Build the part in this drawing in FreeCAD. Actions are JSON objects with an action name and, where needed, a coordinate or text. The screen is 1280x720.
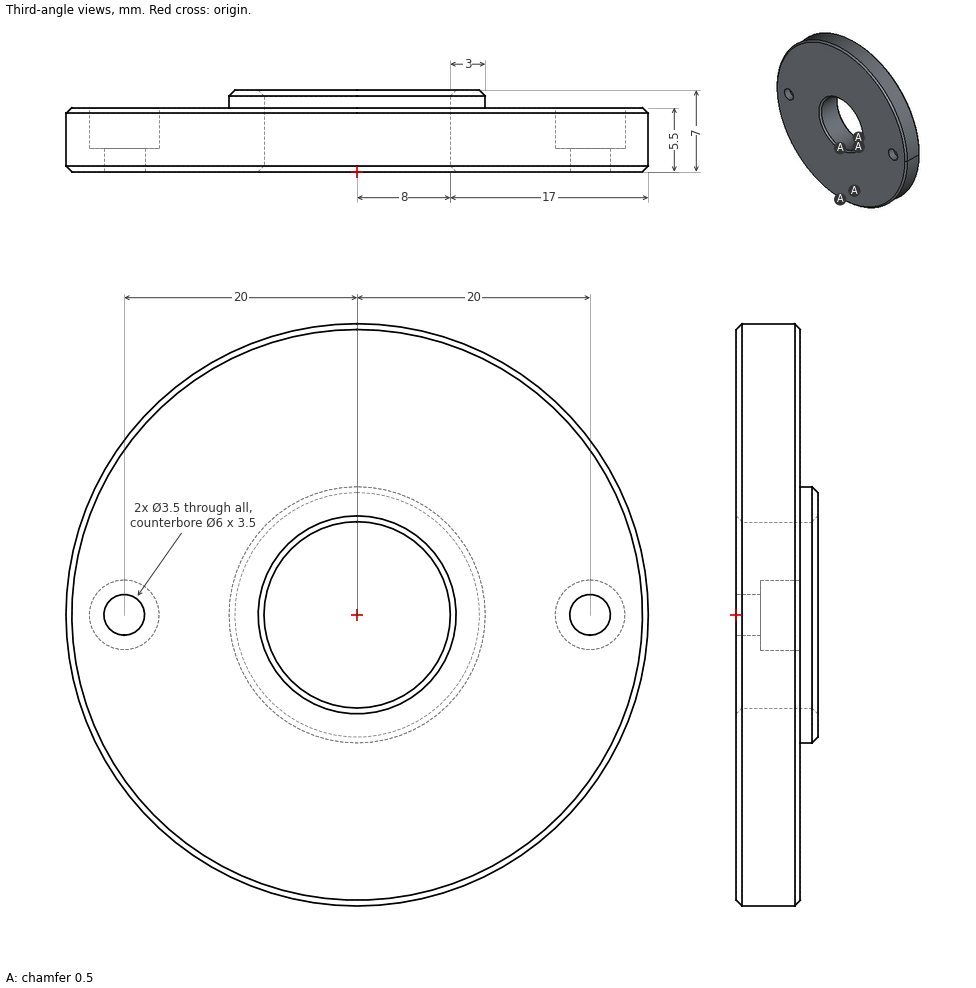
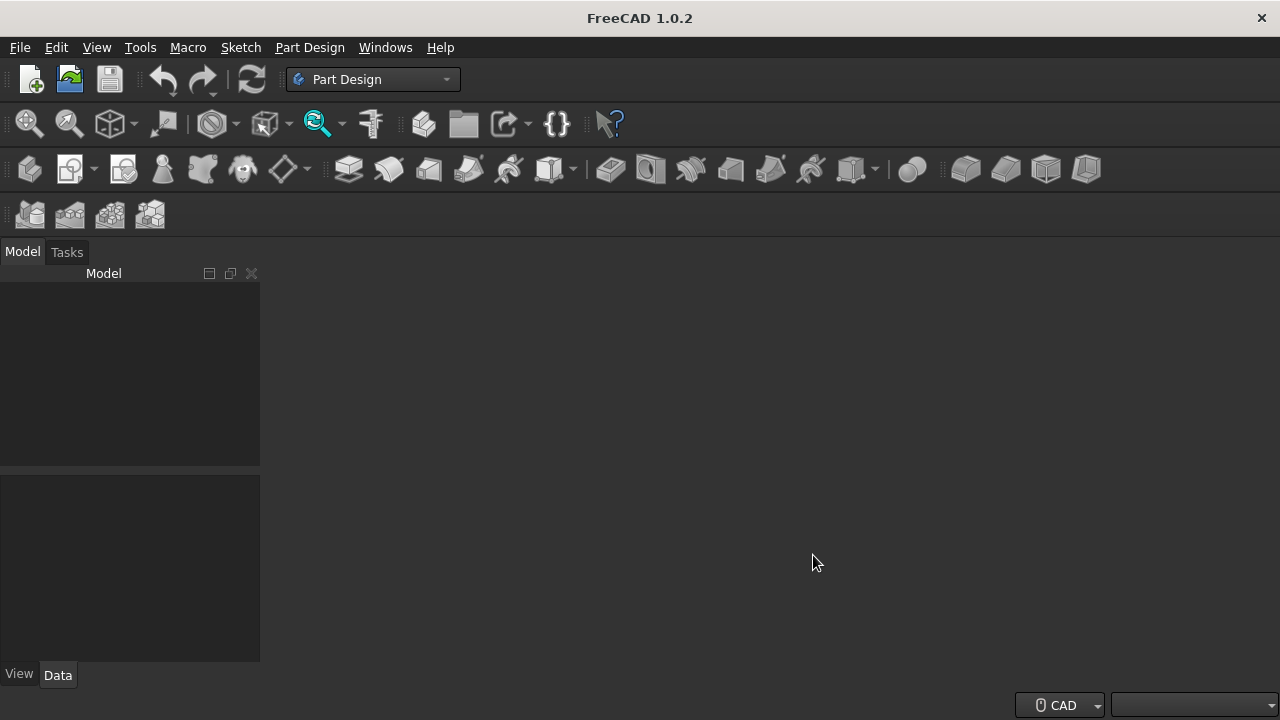
{"action": "left_click", "coordinate": [30, 80]}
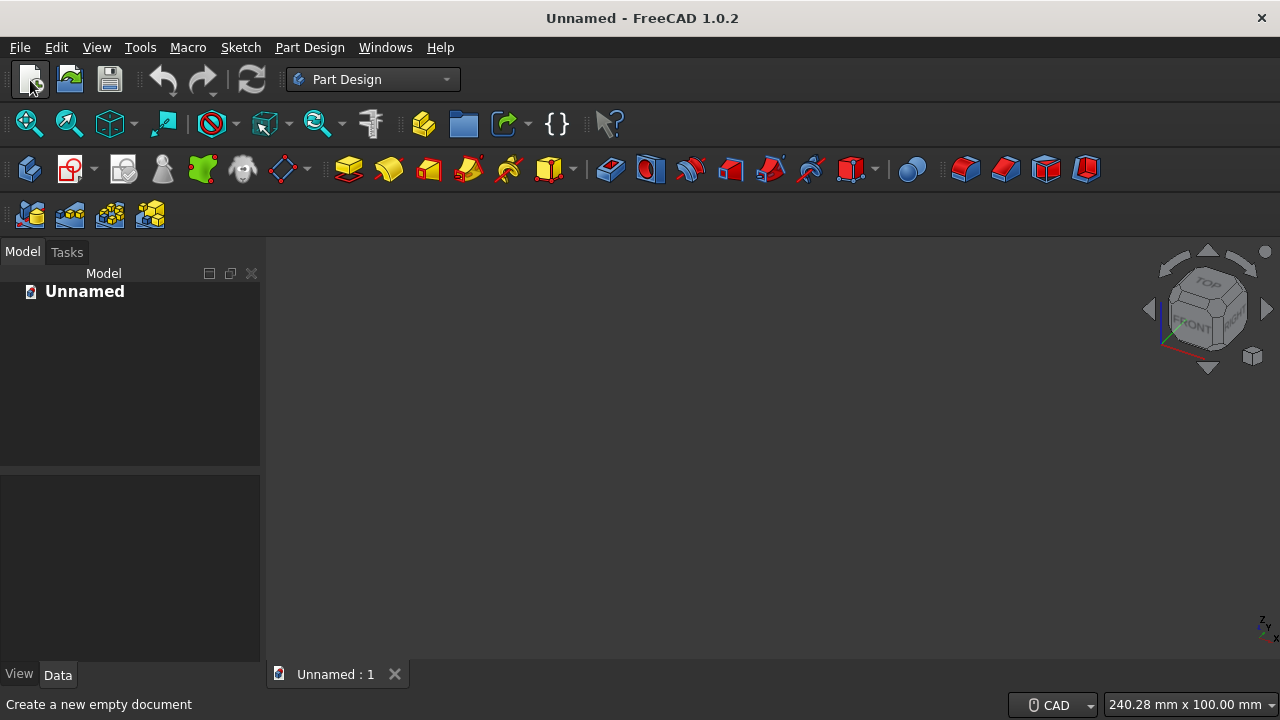
{"action": "left_click", "coordinate": [70, 170]}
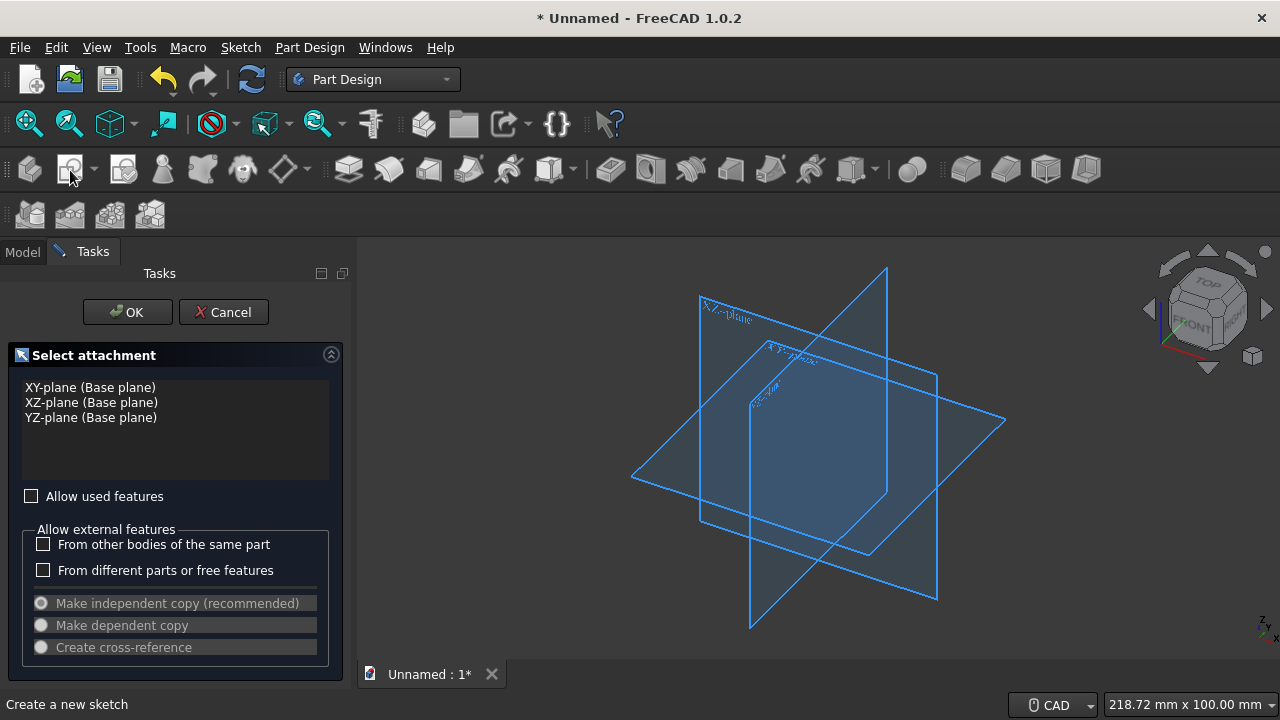
{"action": "left_click", "coordinate": [82, 388]}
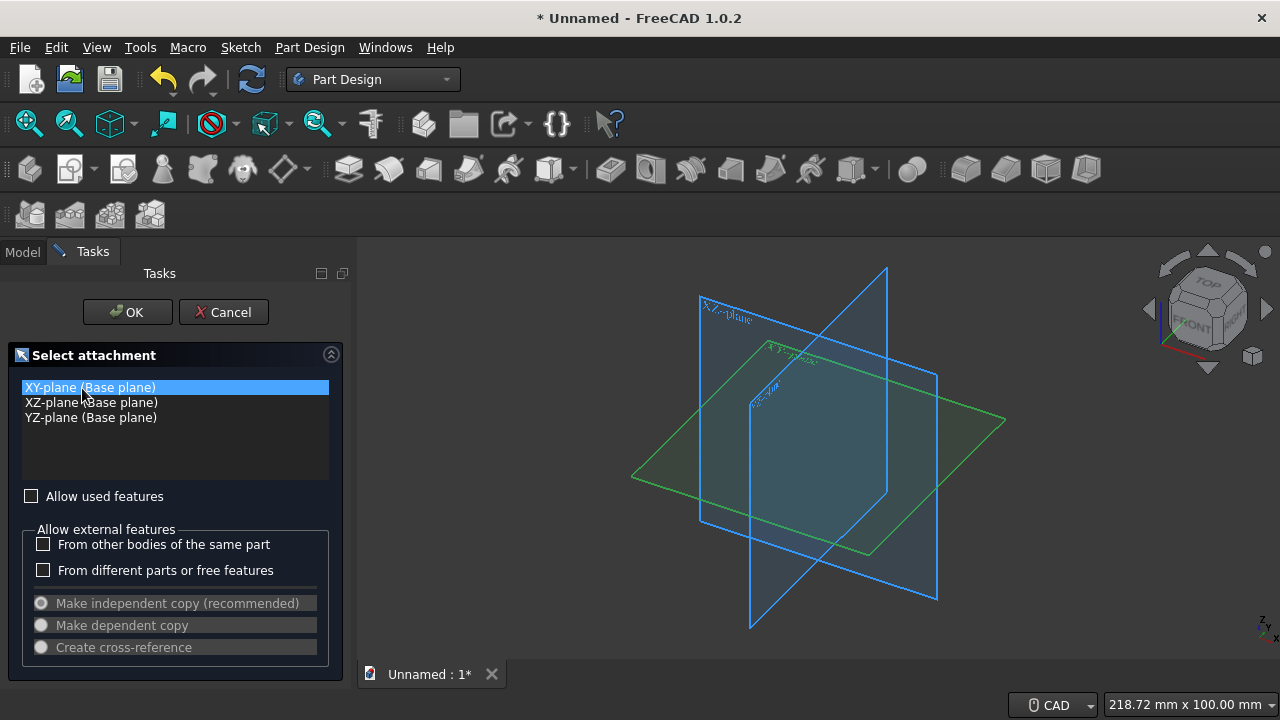
{"action": "left_click", "coordinate": [128, 312]}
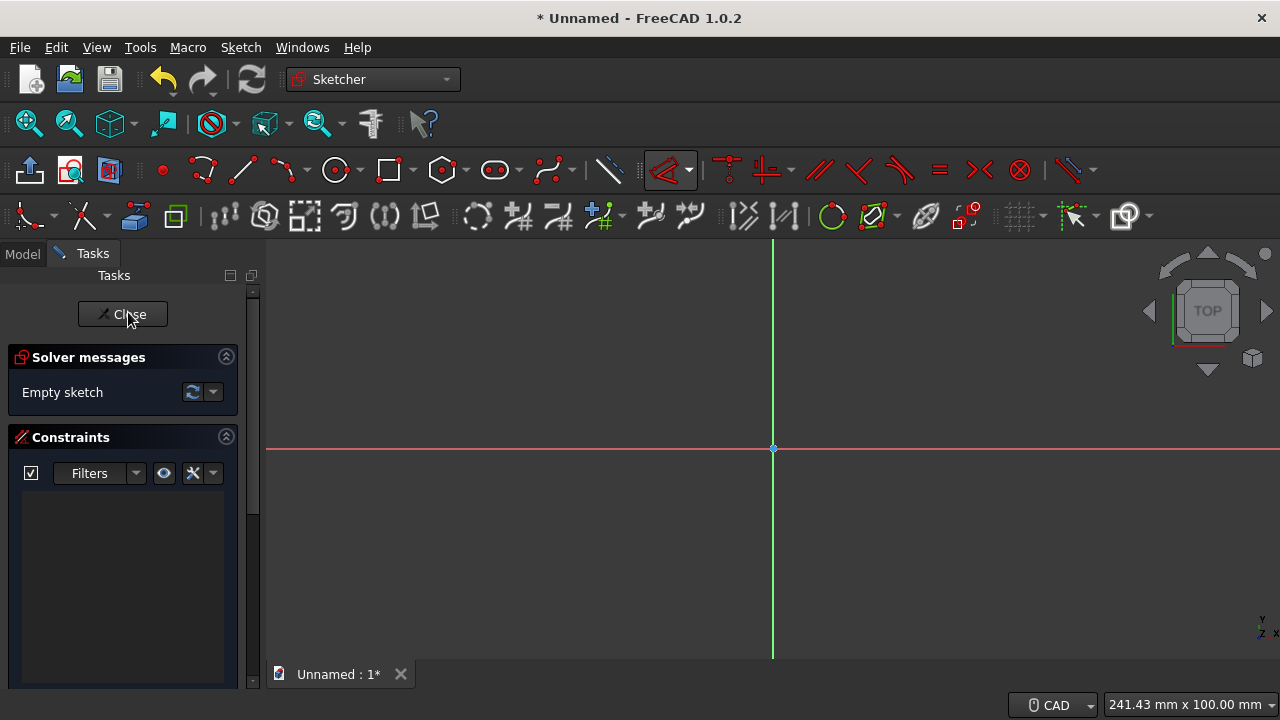
{"action": "scroll", "coordinate": [849, 431], "scroll_direction": "up", "scroll_amount": 9}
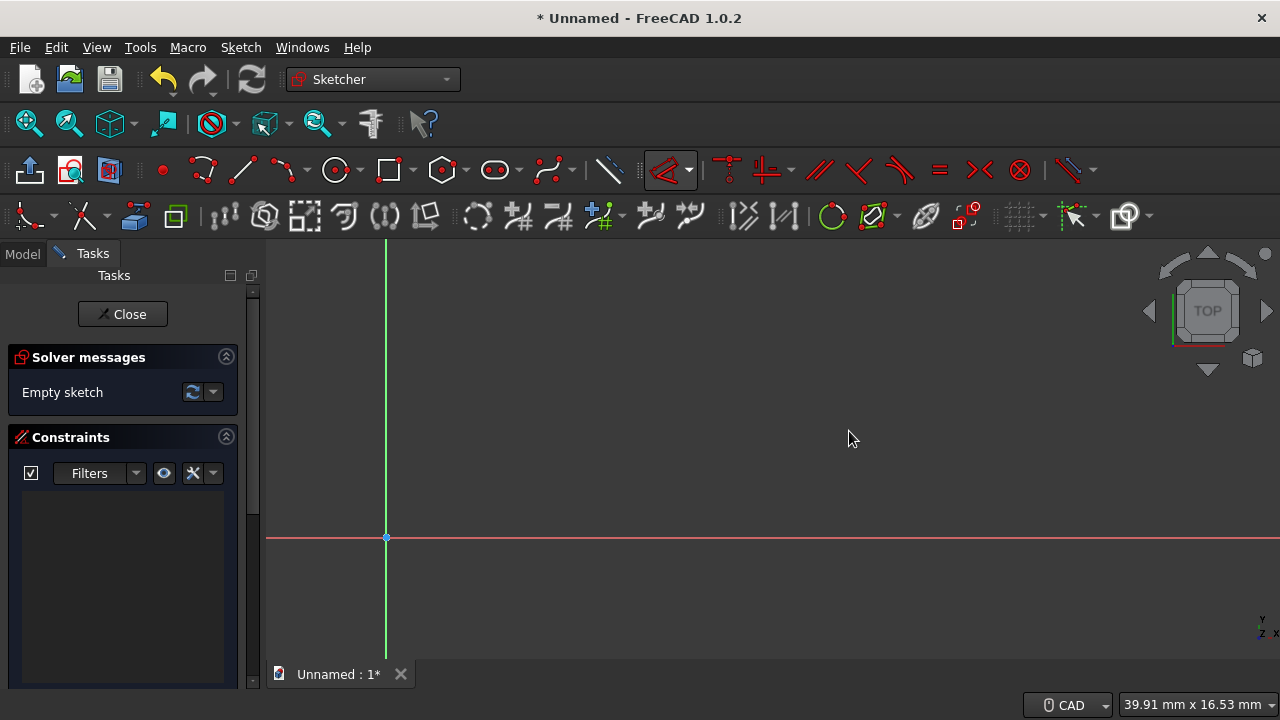
{"action": "key", "text": "g m"}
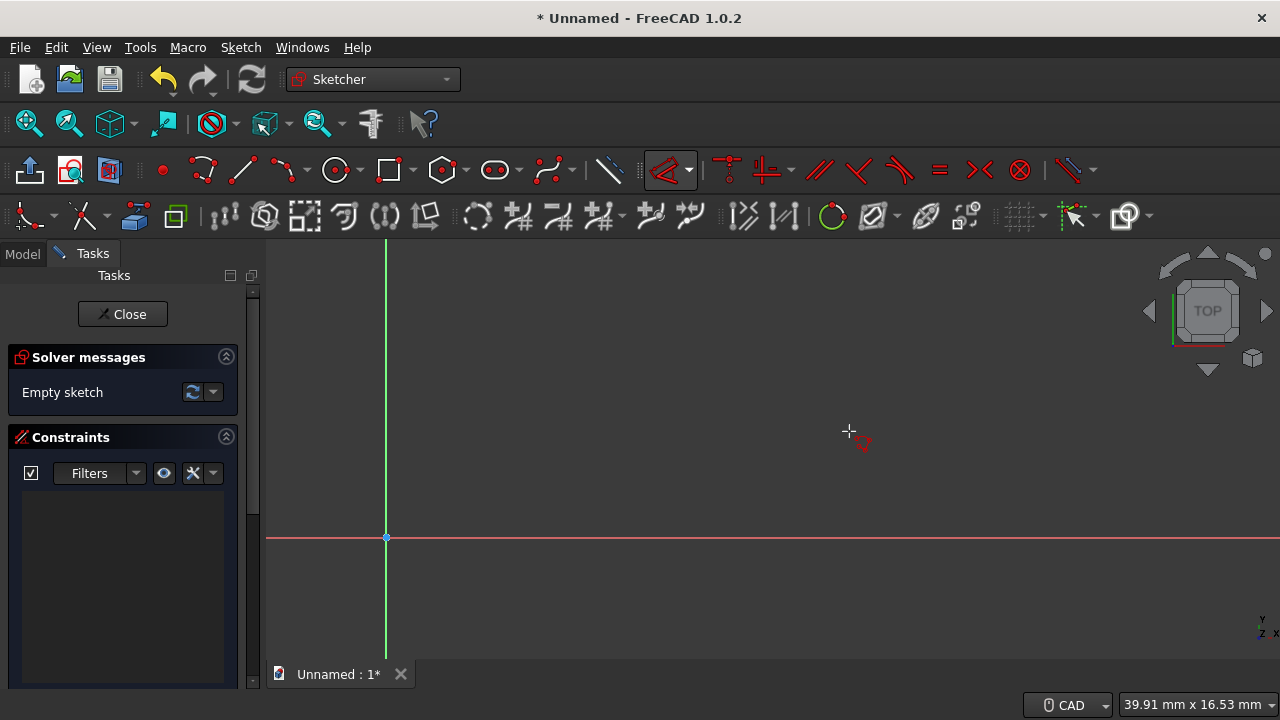
{"action": "left_click", "coordinate": [590, 538]}
{"action": "left_click", "coordinate": [1022, 529]}
{"action": "left_click", "coordinate": [1022, 398]}
{"action": "left_click", "coordinate": [666, 398]}
{"action": "left_click", "coordinate": [666, 360]}
{"action": "left_click", "coordinate": [590, 360]}
{"action": "left_click", "coordinate": [590, 538]}
{"action": "key", "text": "Escape"}
{"action": "key", "text": "Escape"}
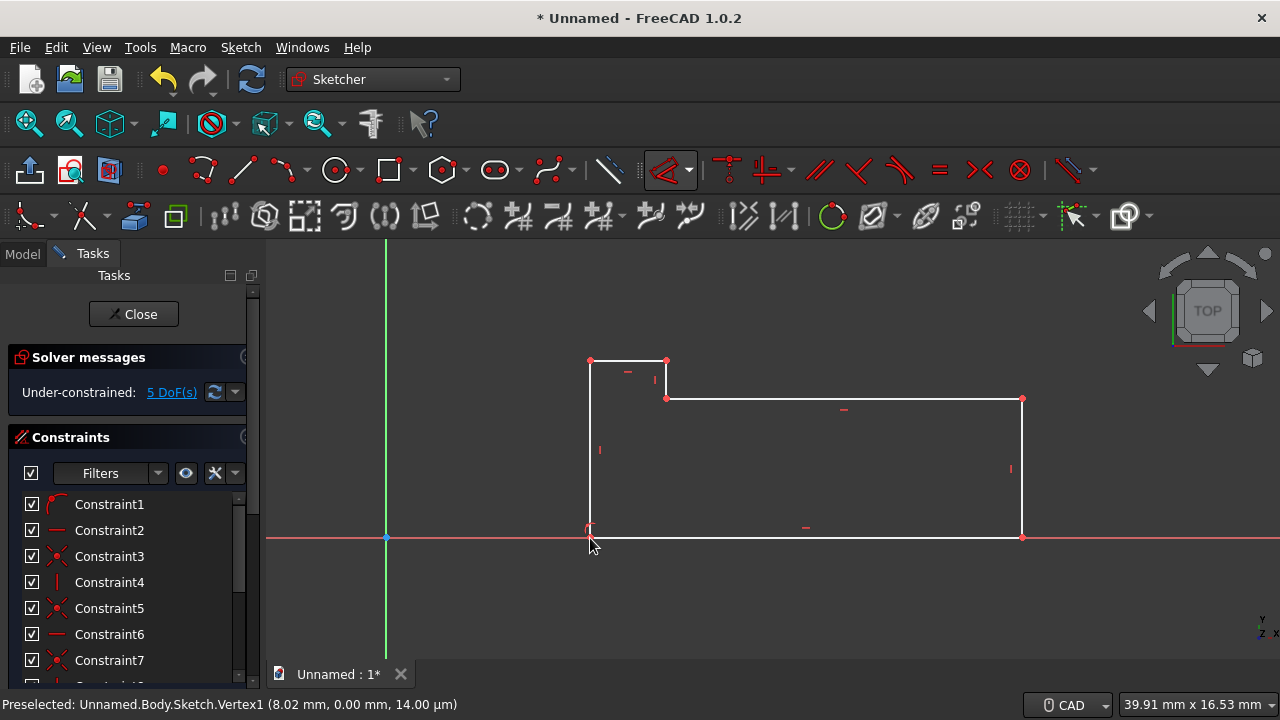
{"action": "left_click", "coordinate": [643, 361]}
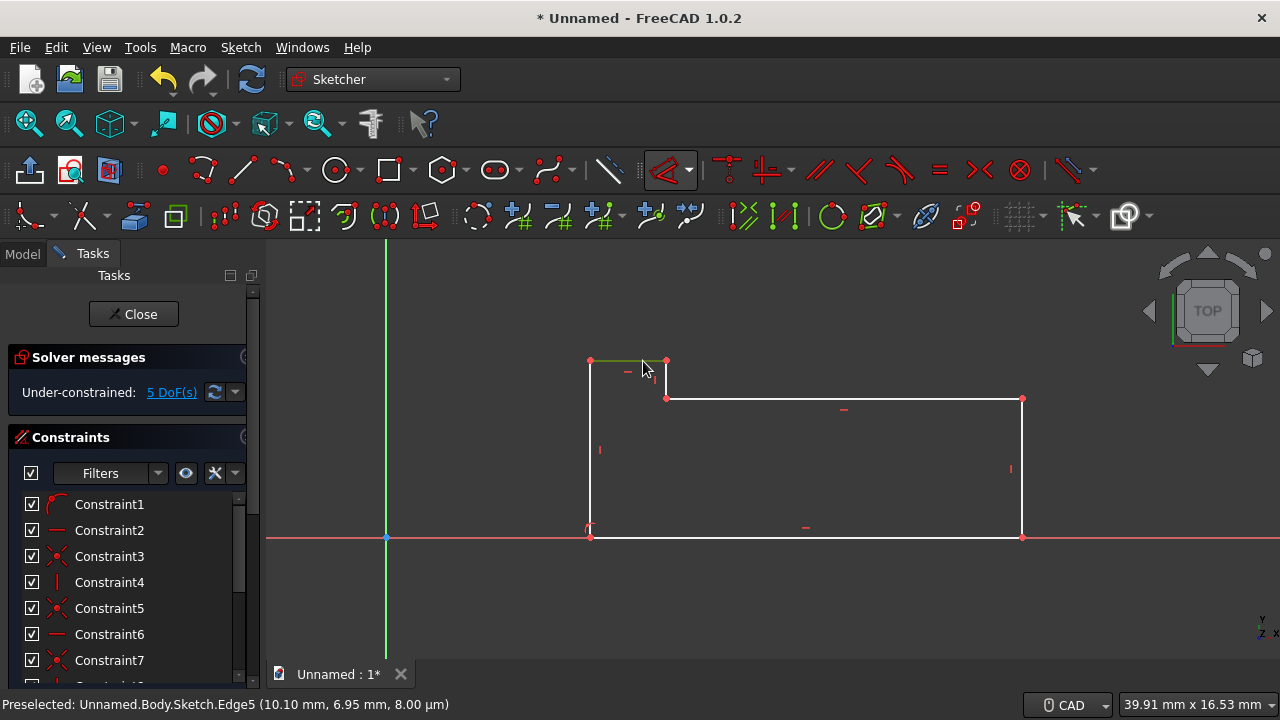
{"action": "key", "text": "l"}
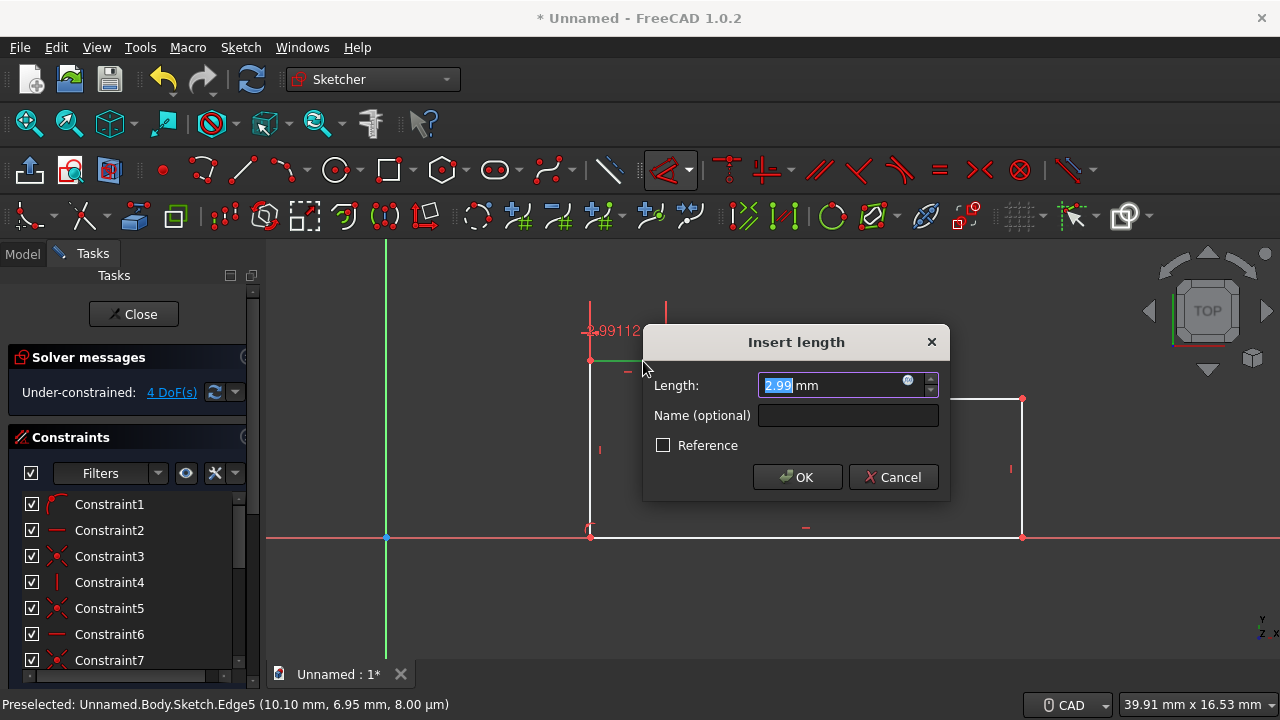
{"action": "type", "text": "3"}
{"action": "key", "text": "Return"}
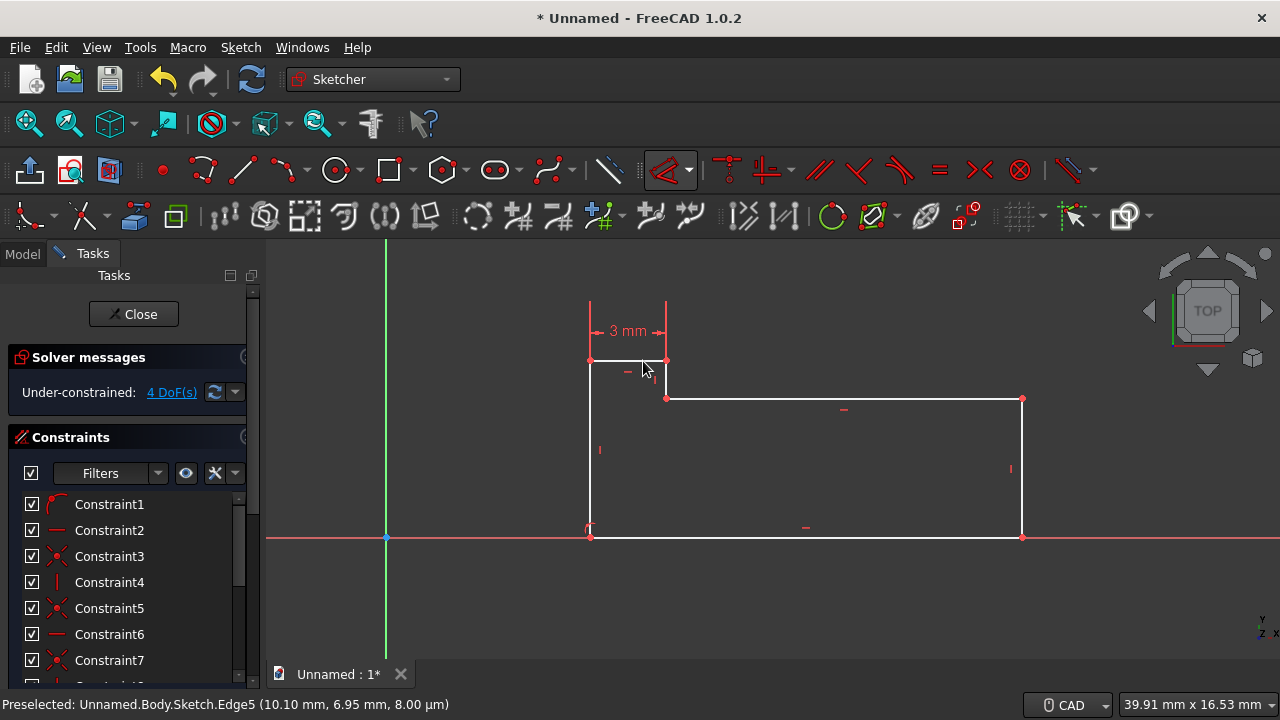
{"action": "left_click", "coordinate": [590, 414]}